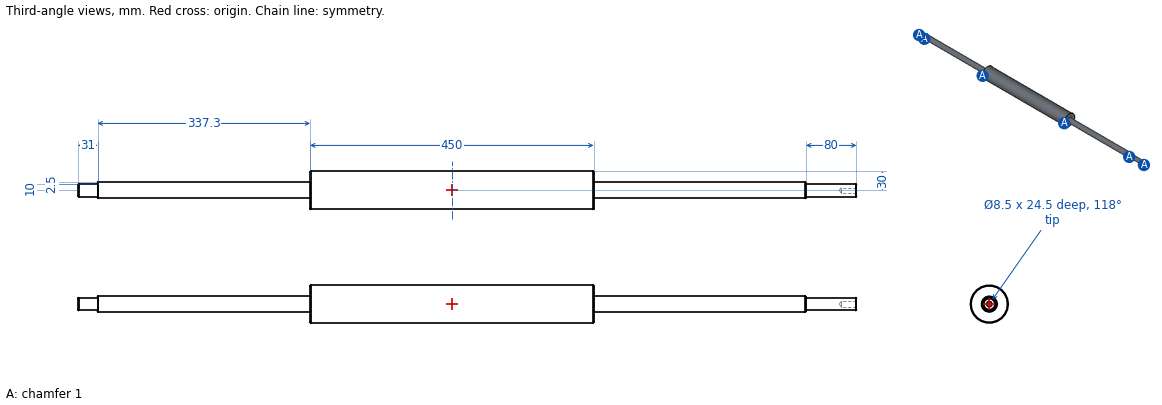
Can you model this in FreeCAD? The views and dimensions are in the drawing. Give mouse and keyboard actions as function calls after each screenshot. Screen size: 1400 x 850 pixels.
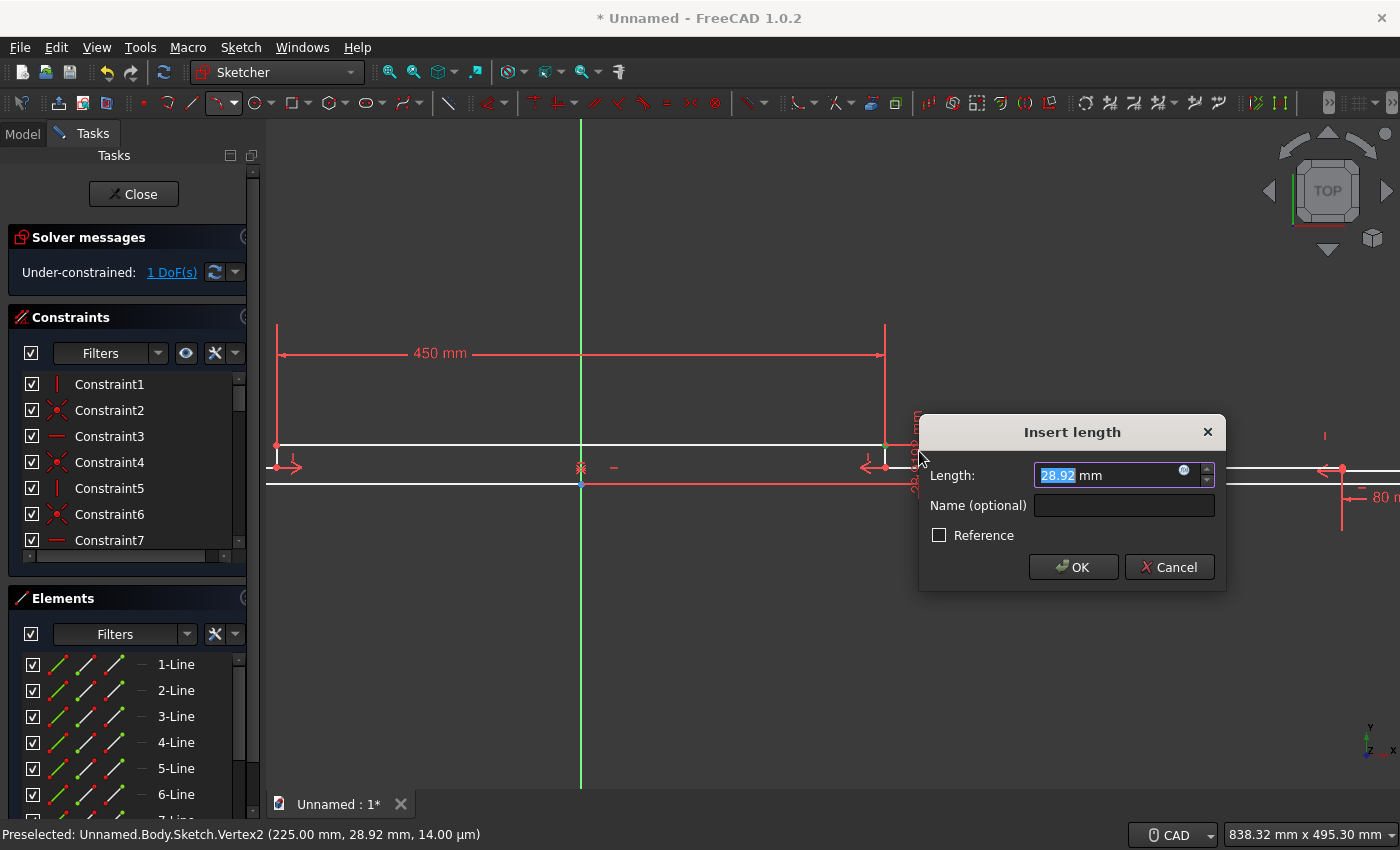
text(30)
key(Return)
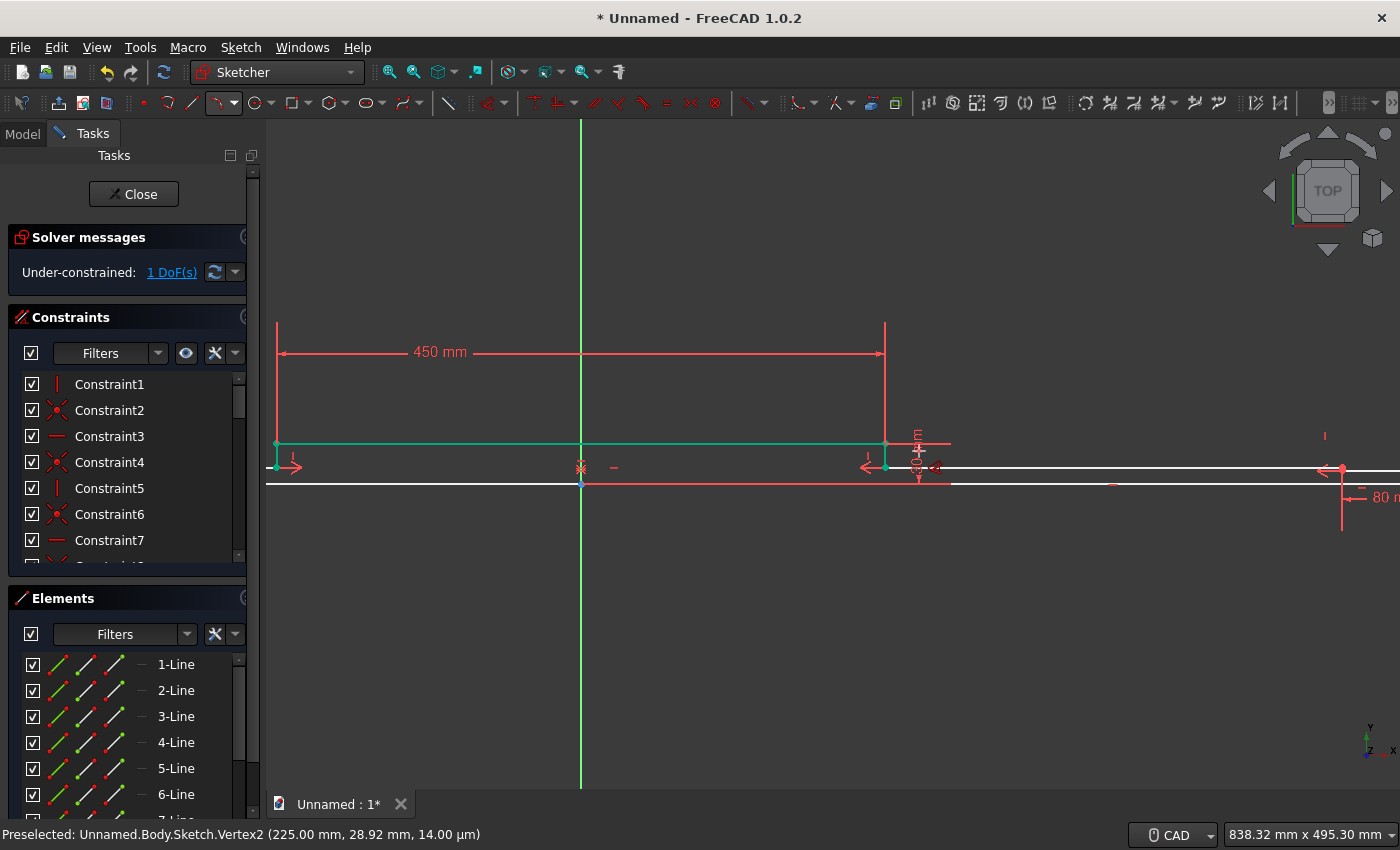
scroll(852, 448, down, 5)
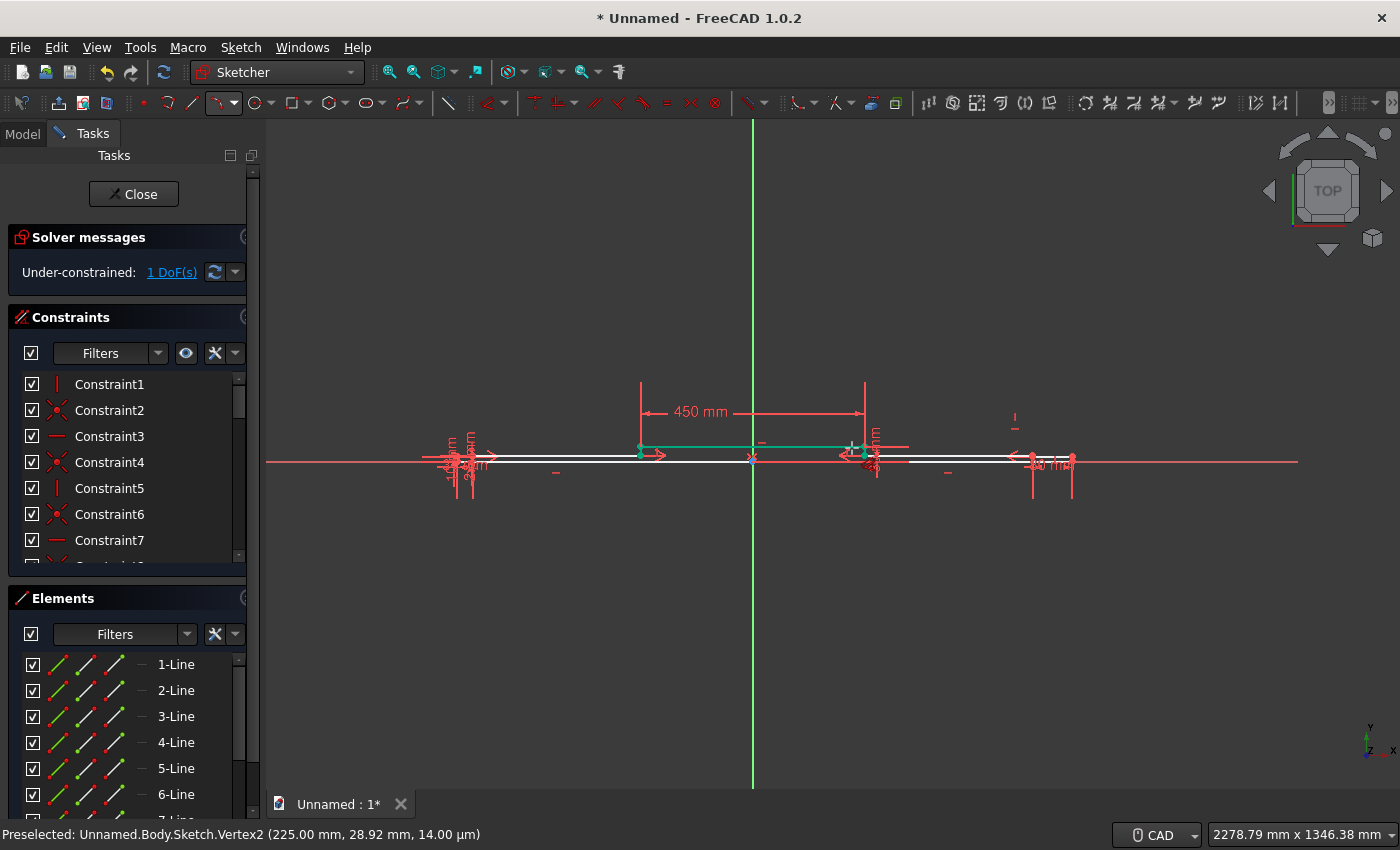
scroll(590, 456, up, 4)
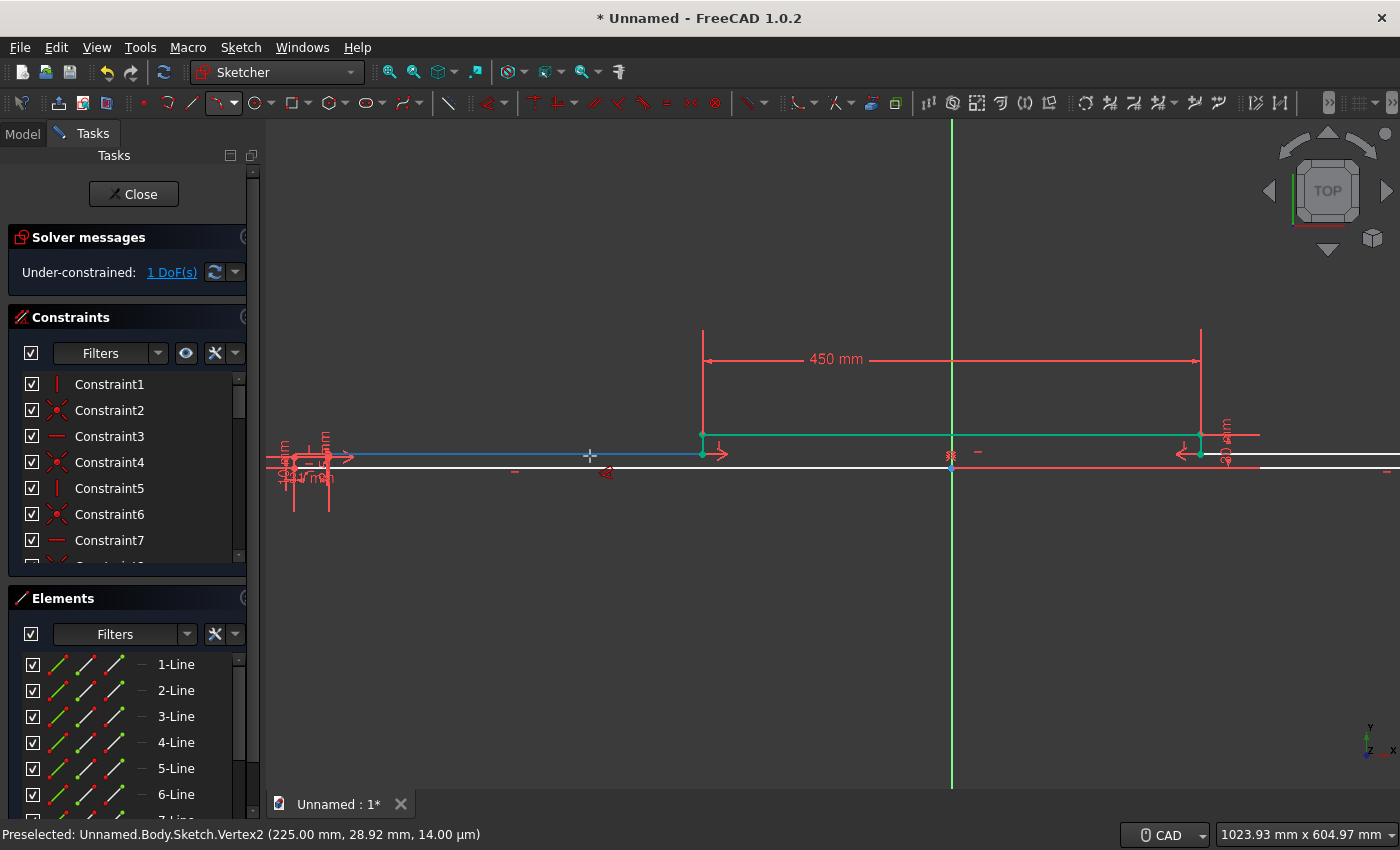
click(590, 454)
click(516, 488)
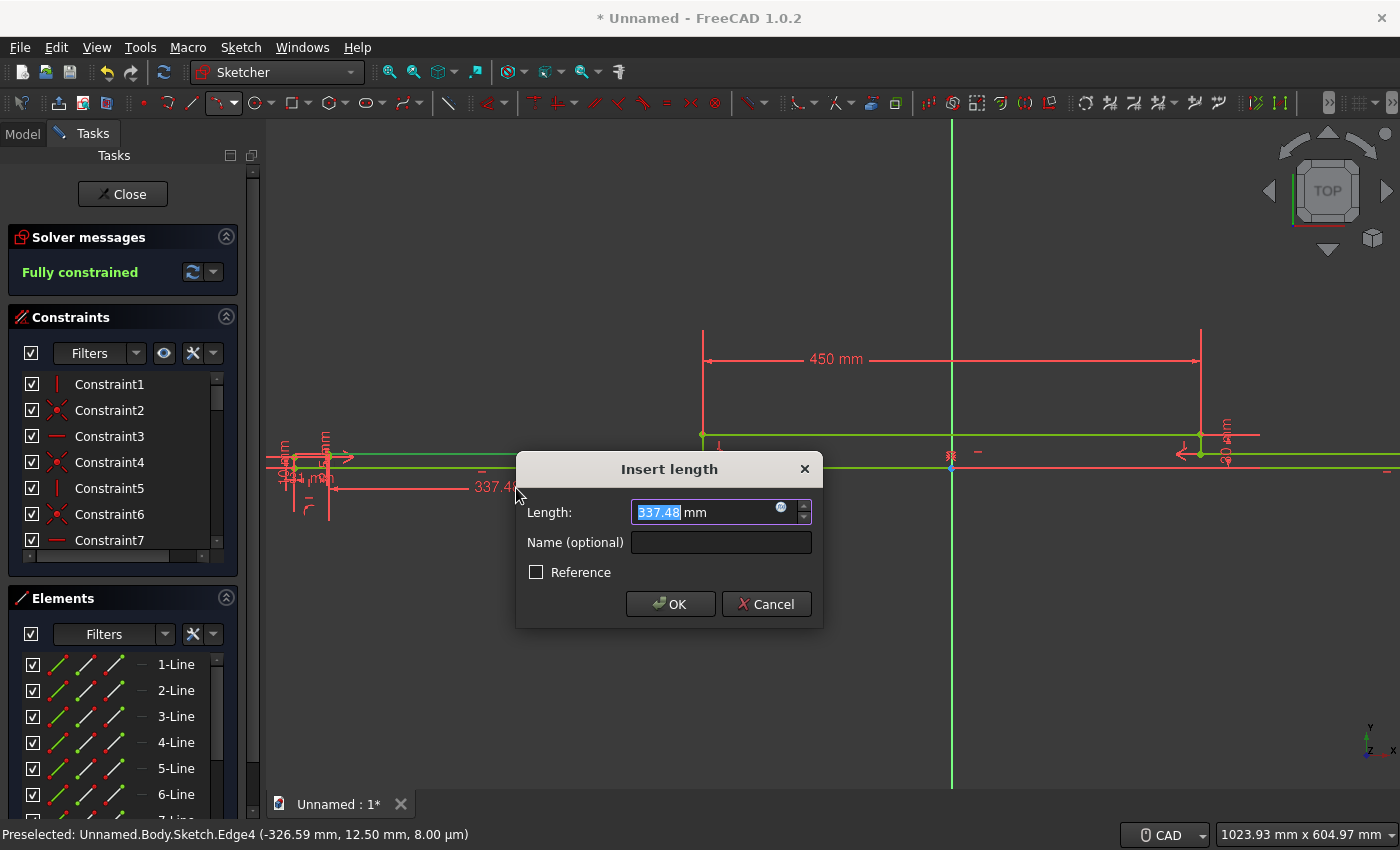
text(337.3)
key(Return)
key(Escape)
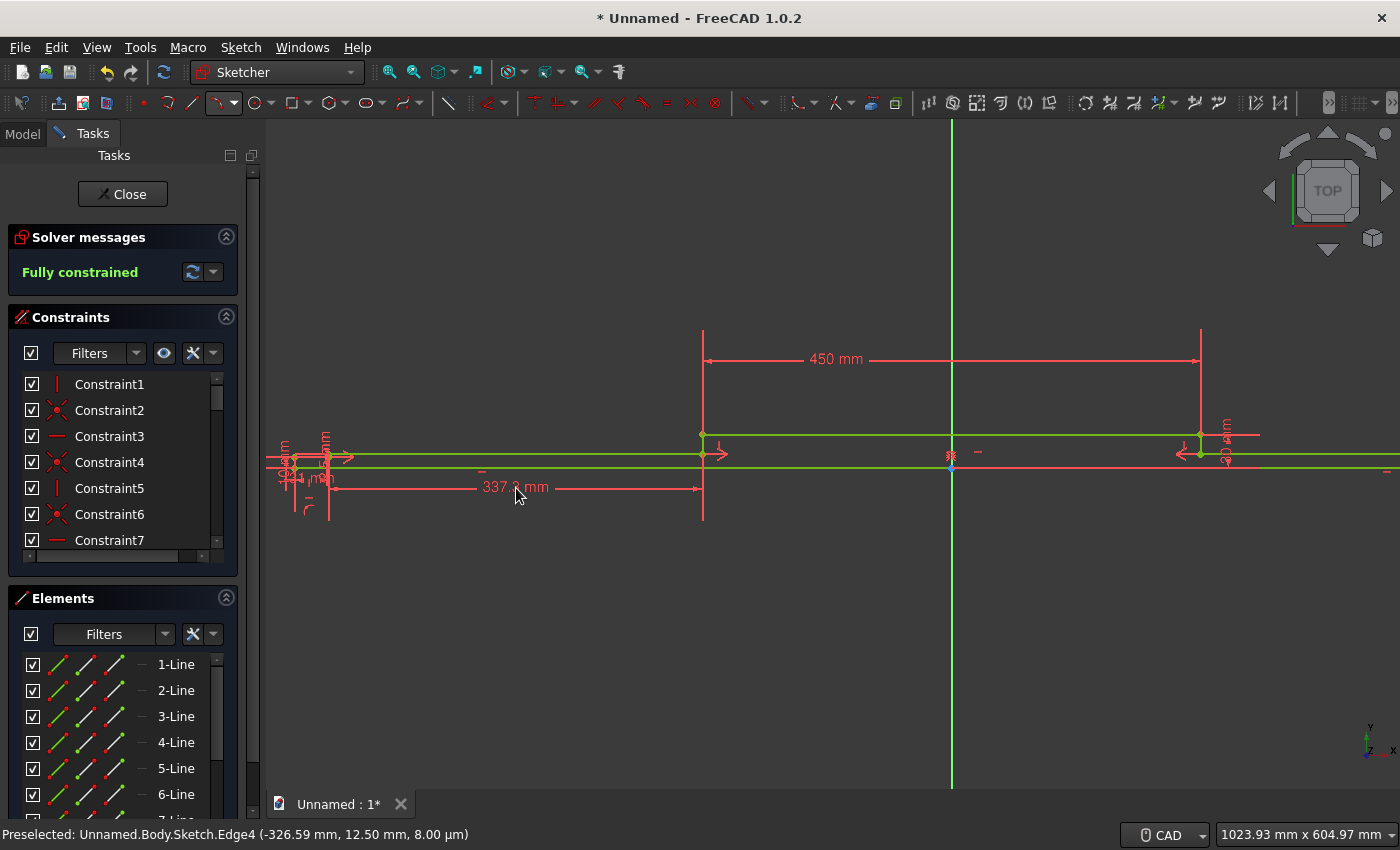
click(123, 194)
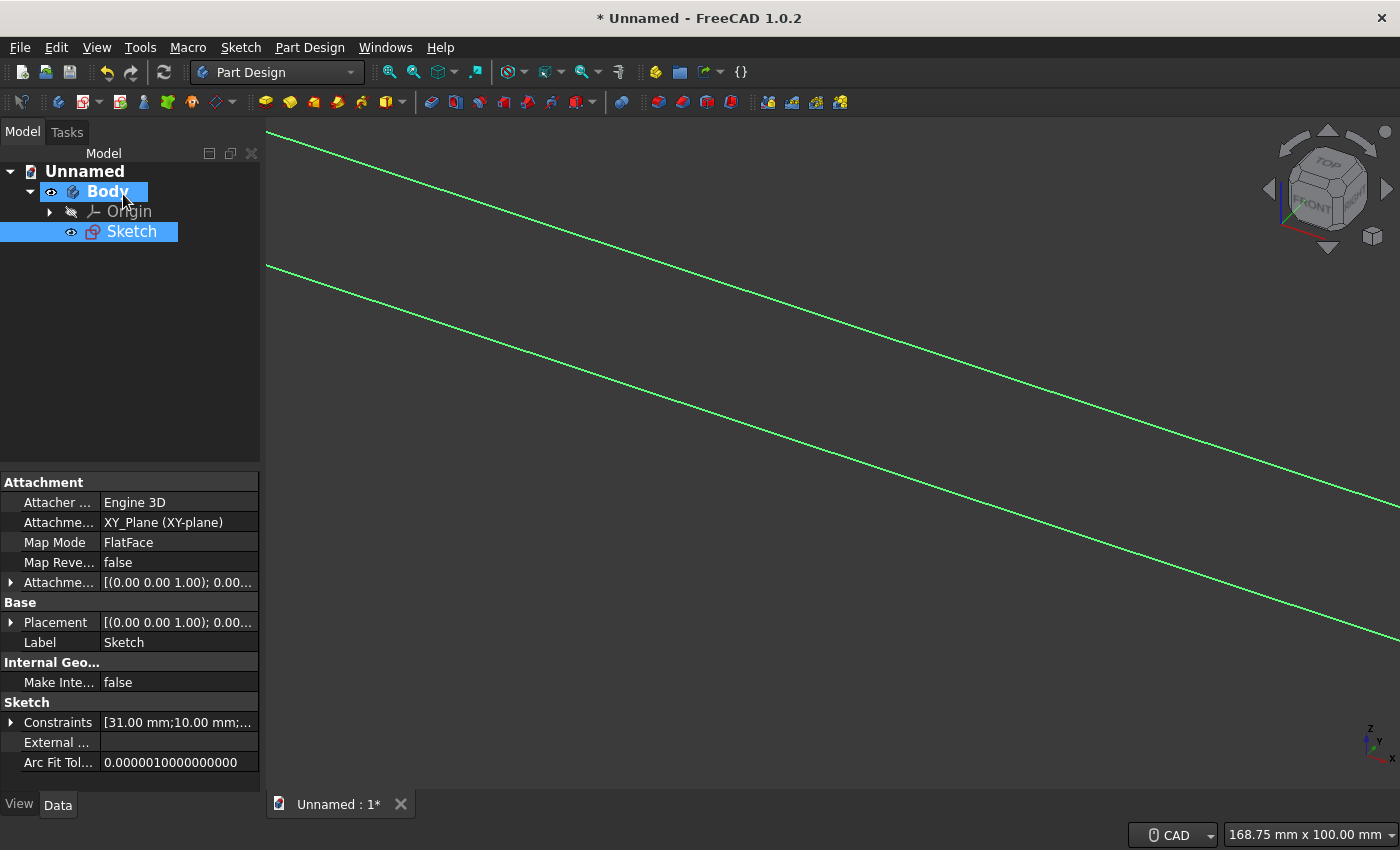
click(290, 102)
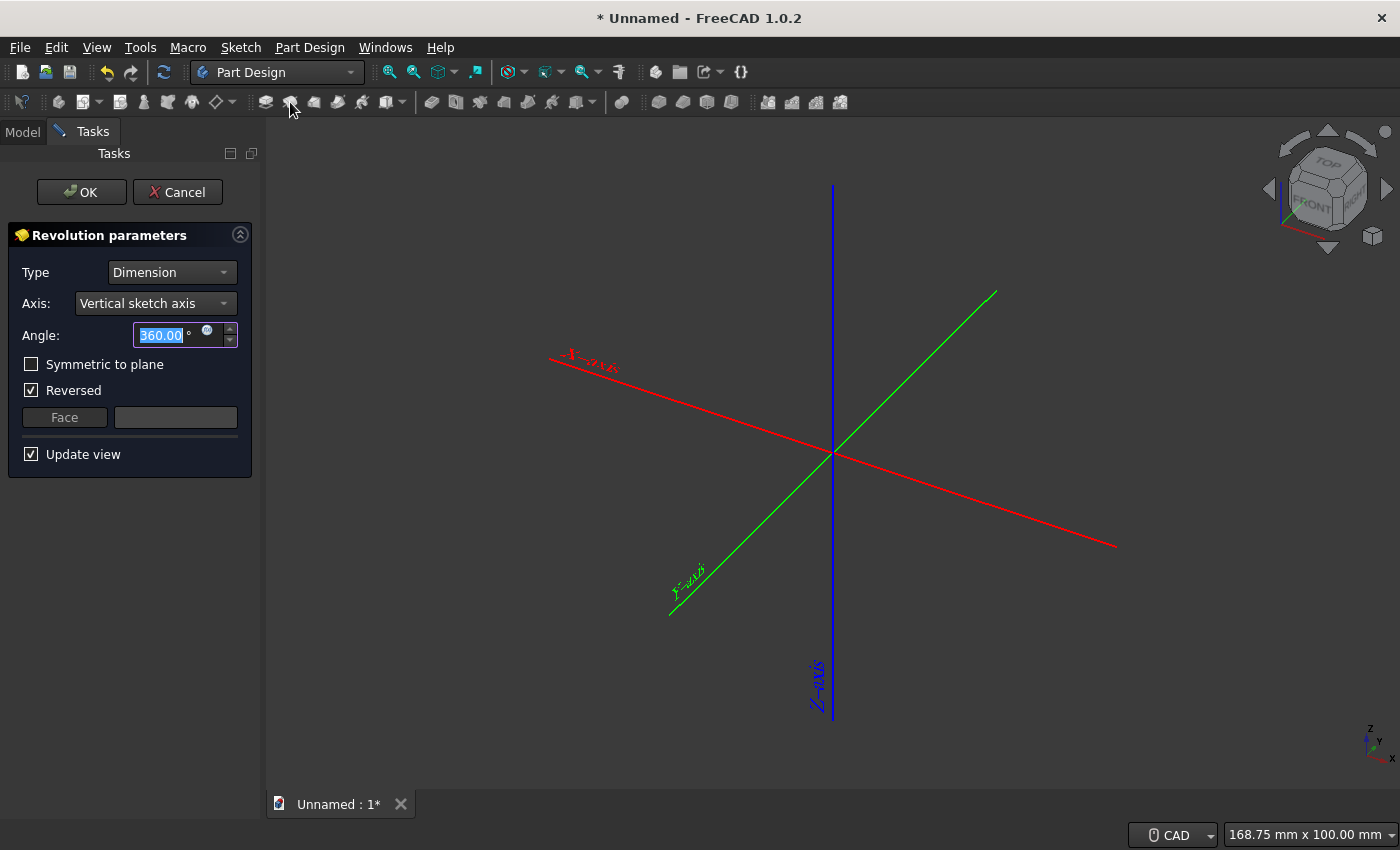
click(156, 304)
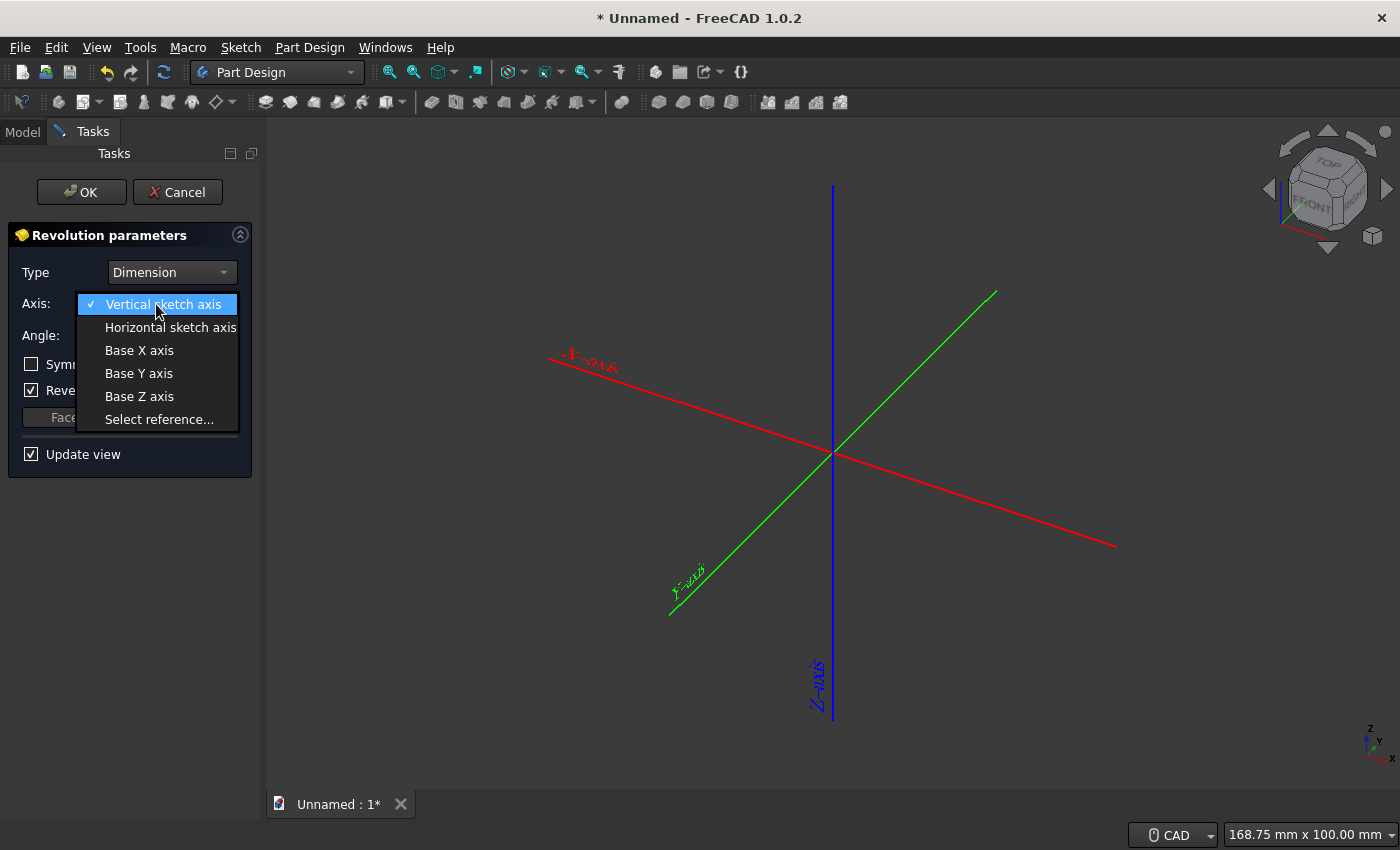
click(156, 328)